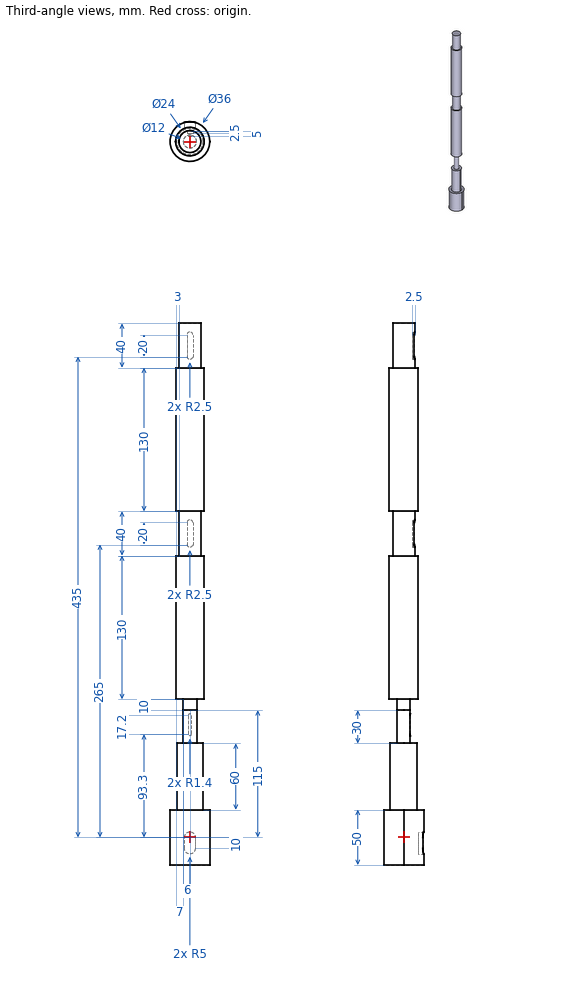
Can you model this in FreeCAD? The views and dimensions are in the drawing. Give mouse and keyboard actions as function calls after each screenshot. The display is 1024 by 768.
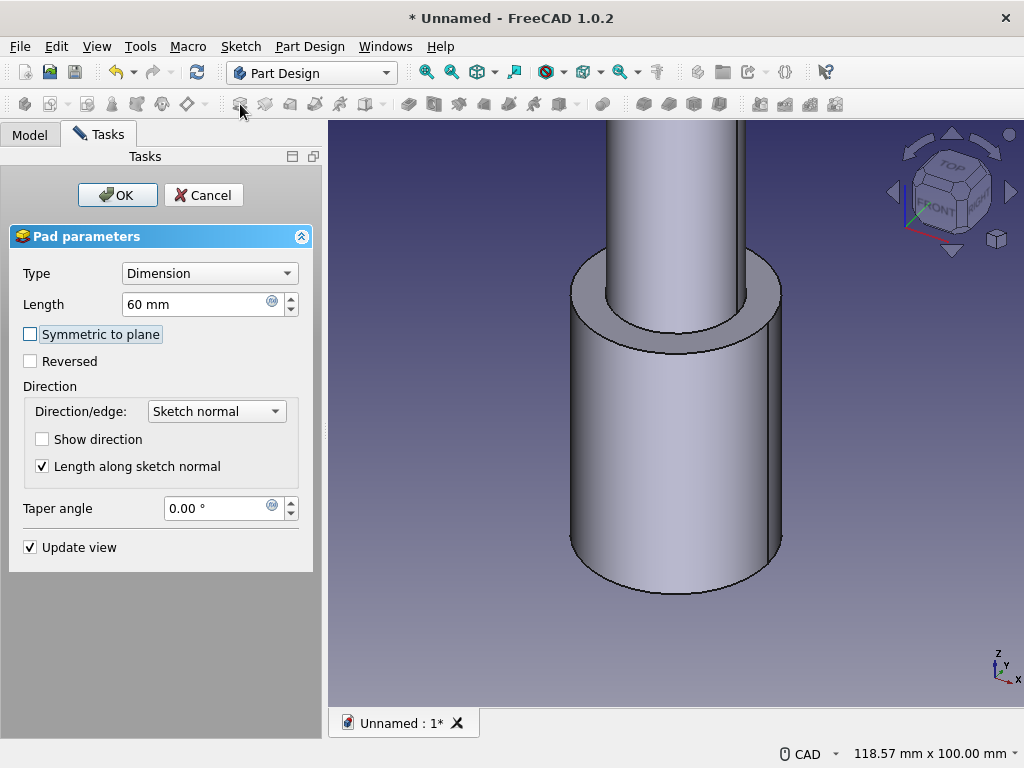
click(118, 195)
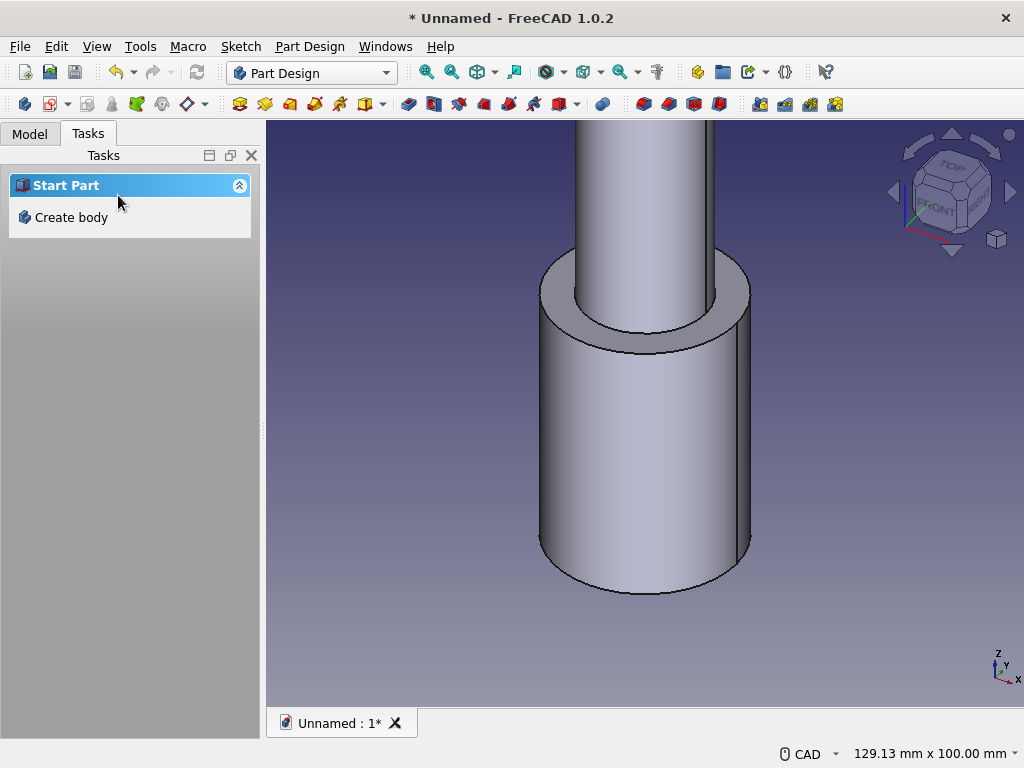
click(427, 72)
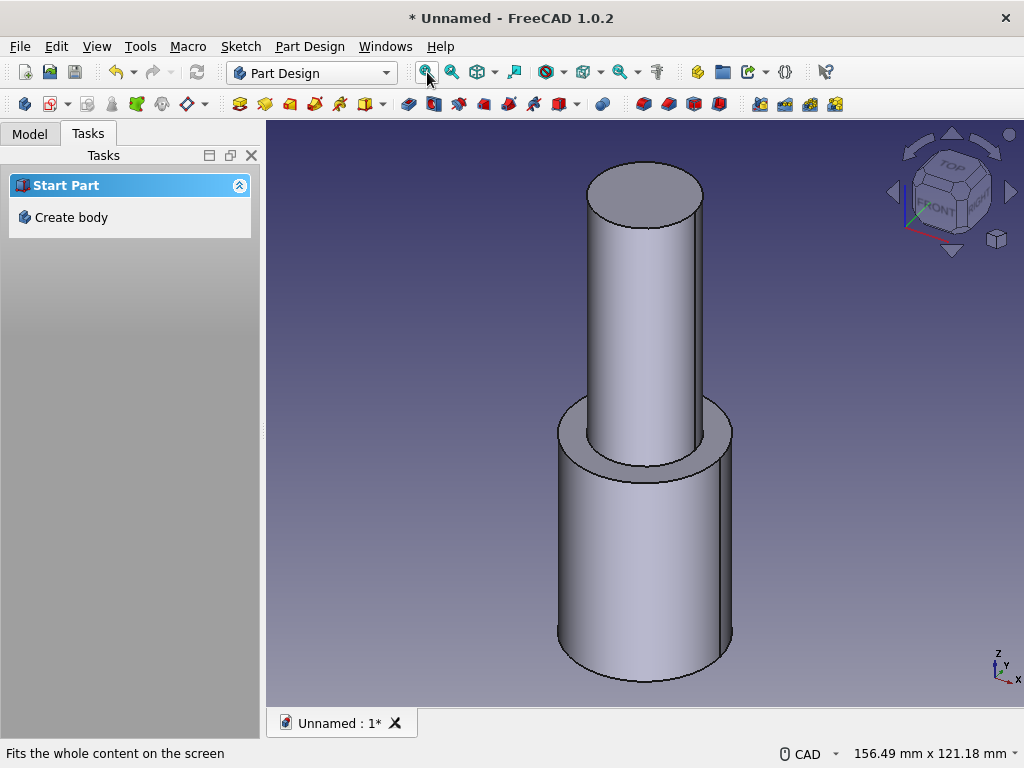
click(645, 194)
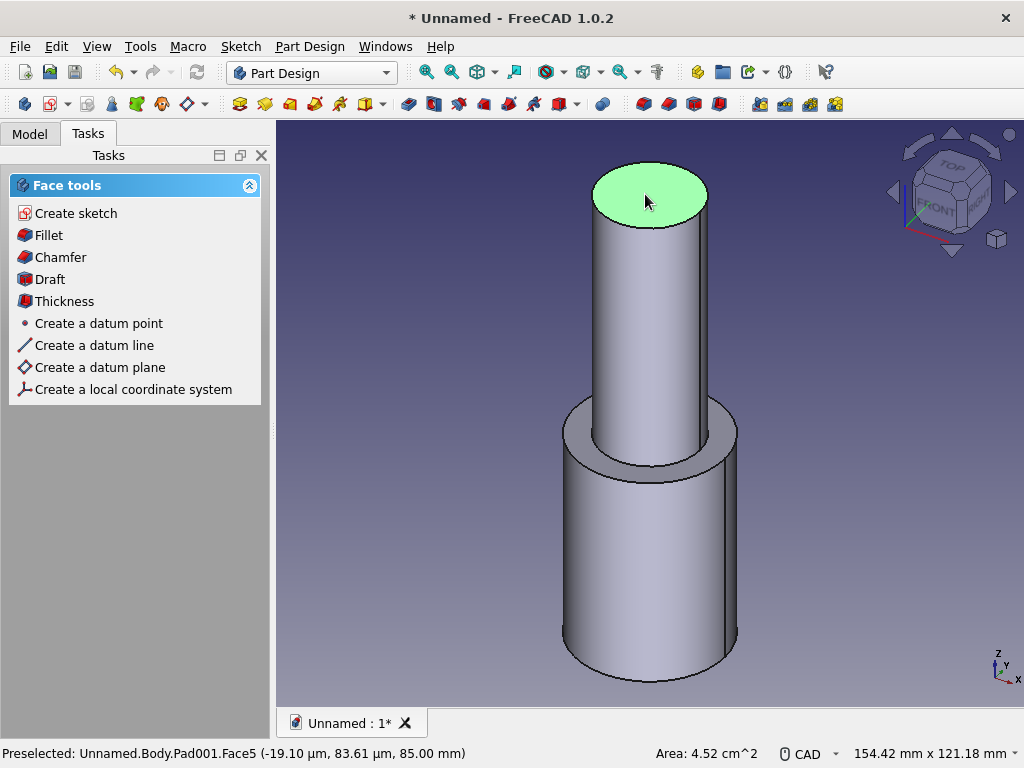
click(50, 104)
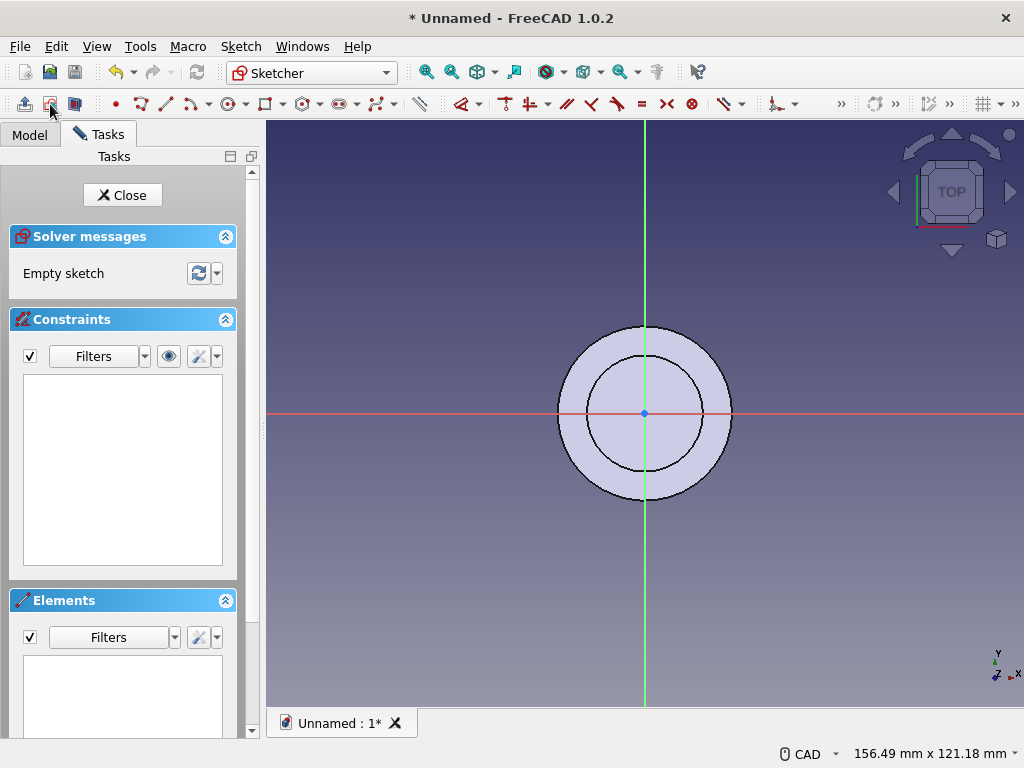
scroll(658, 414, up, 9)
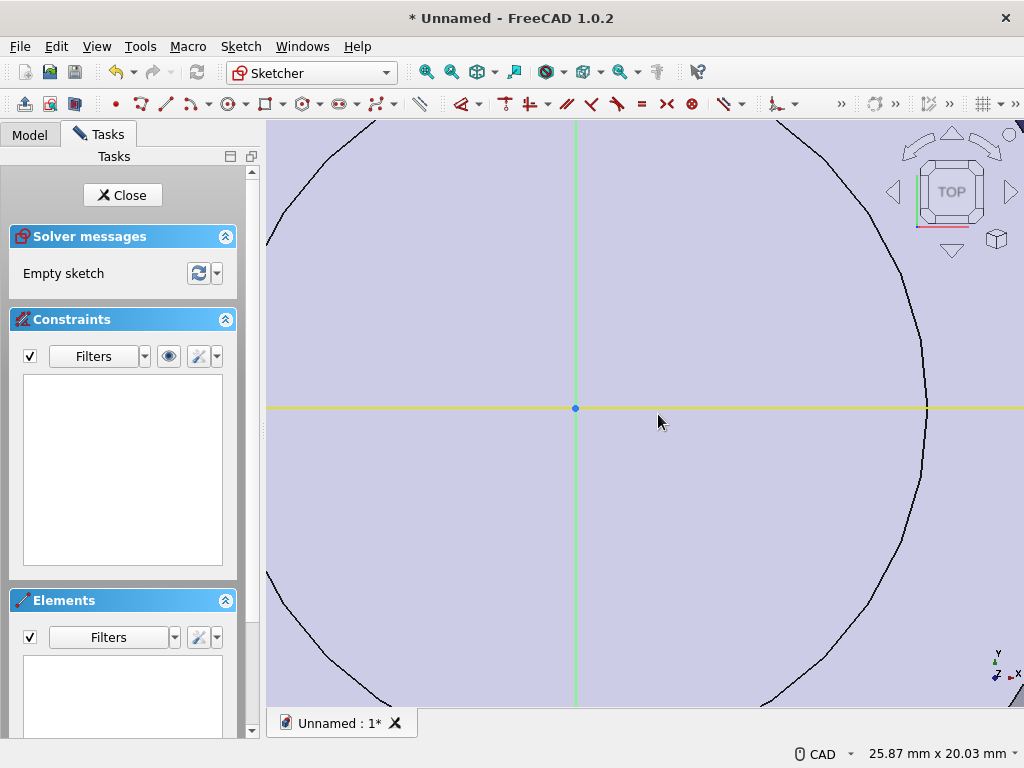
click(228, 104)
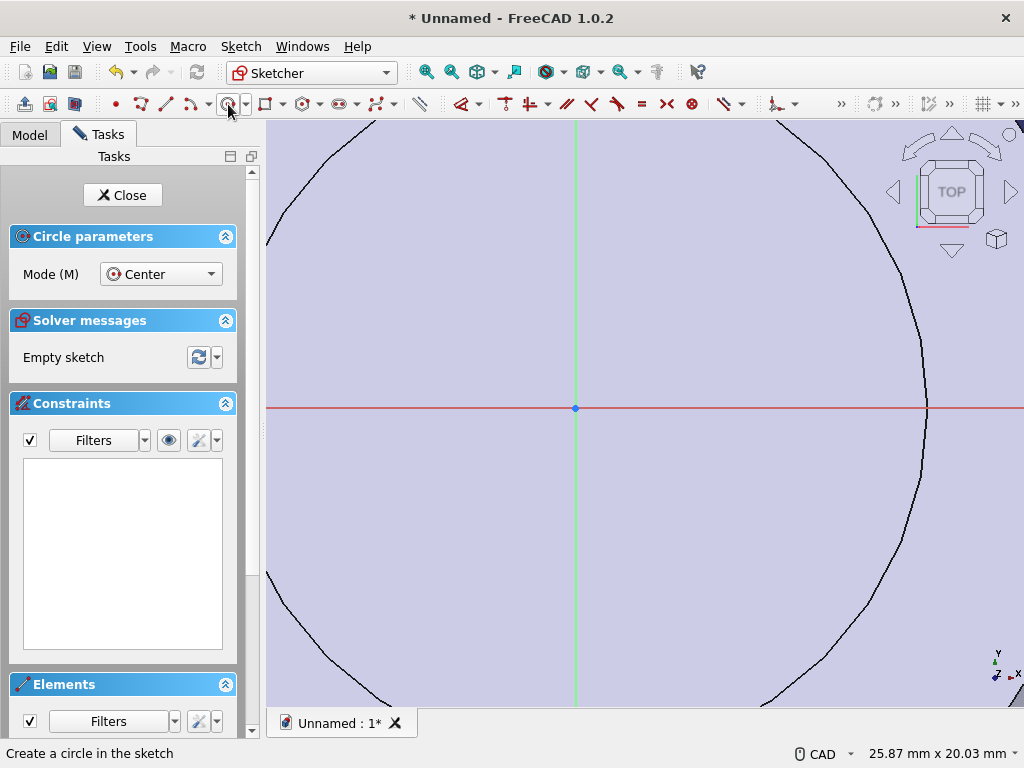
click(576, 408)
click(700, 284)
key(Escape)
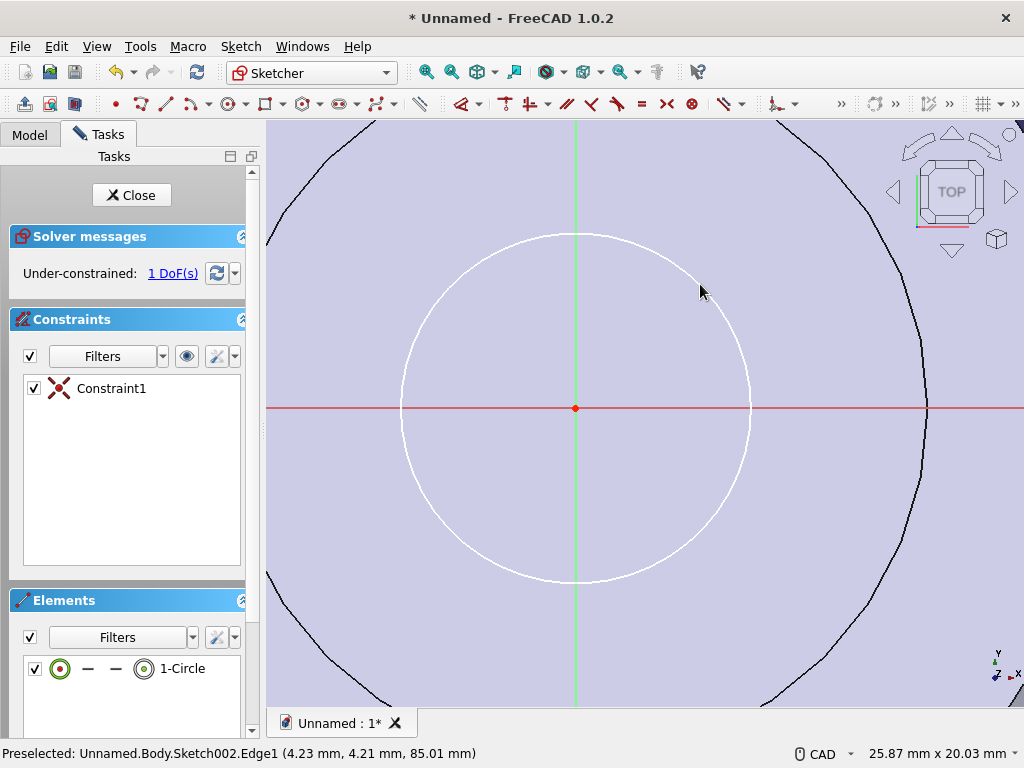
click(460, 104)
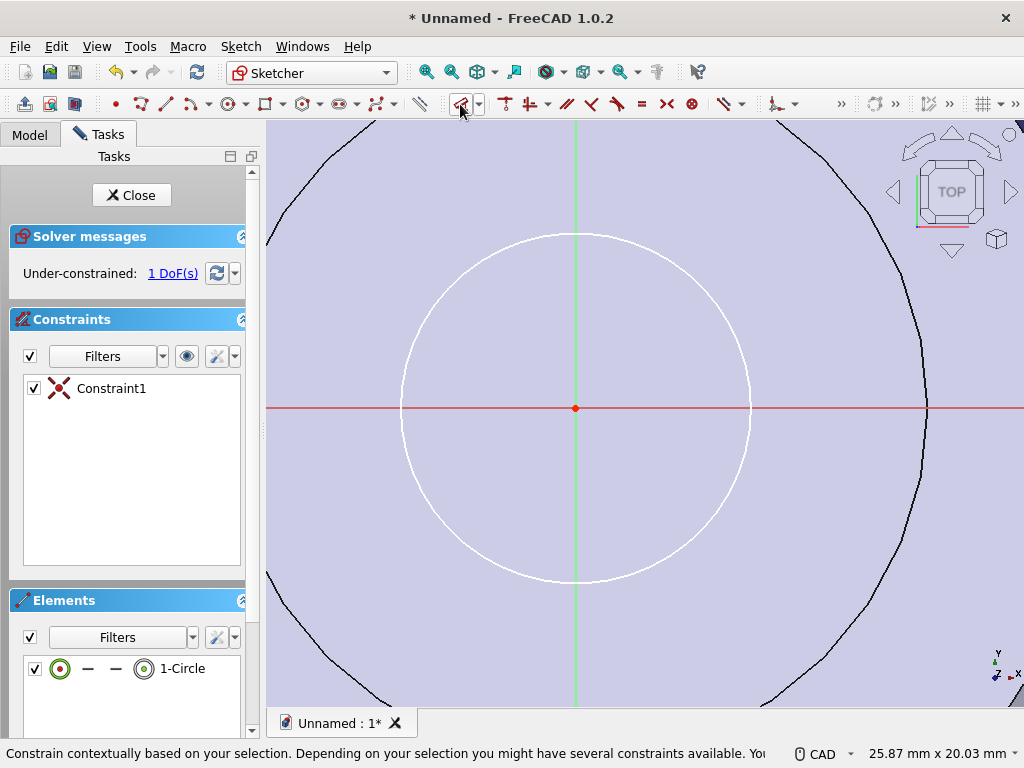
click(699, 284)
click(722, 261)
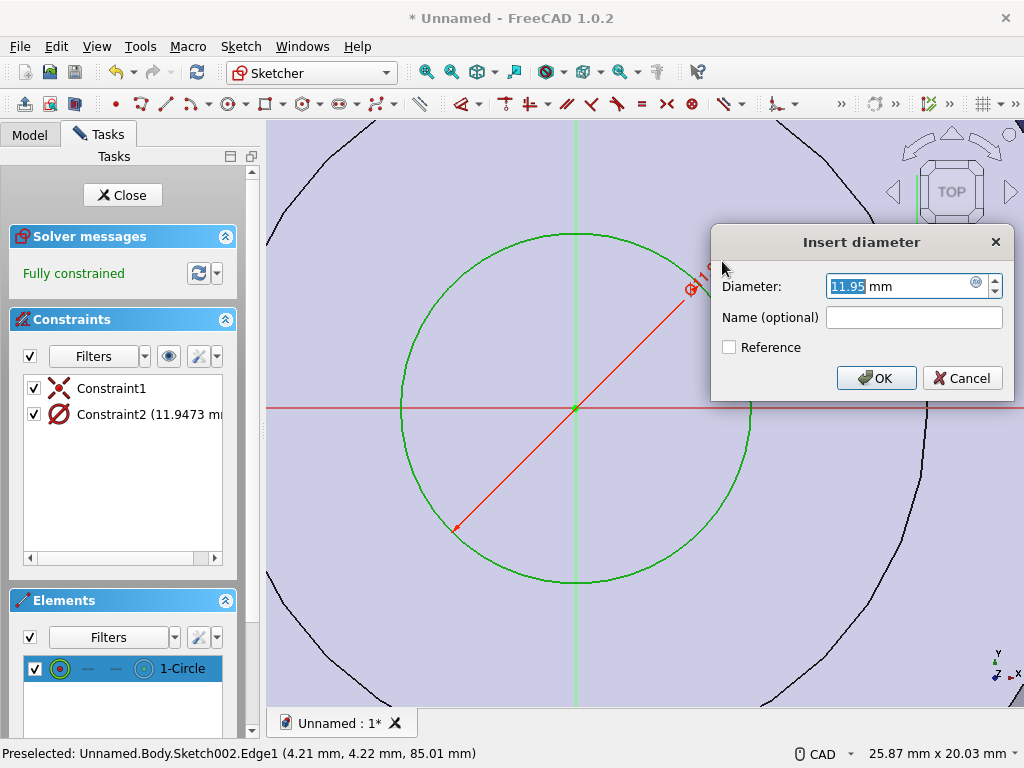
text(12)
key(Return)
key(Escape)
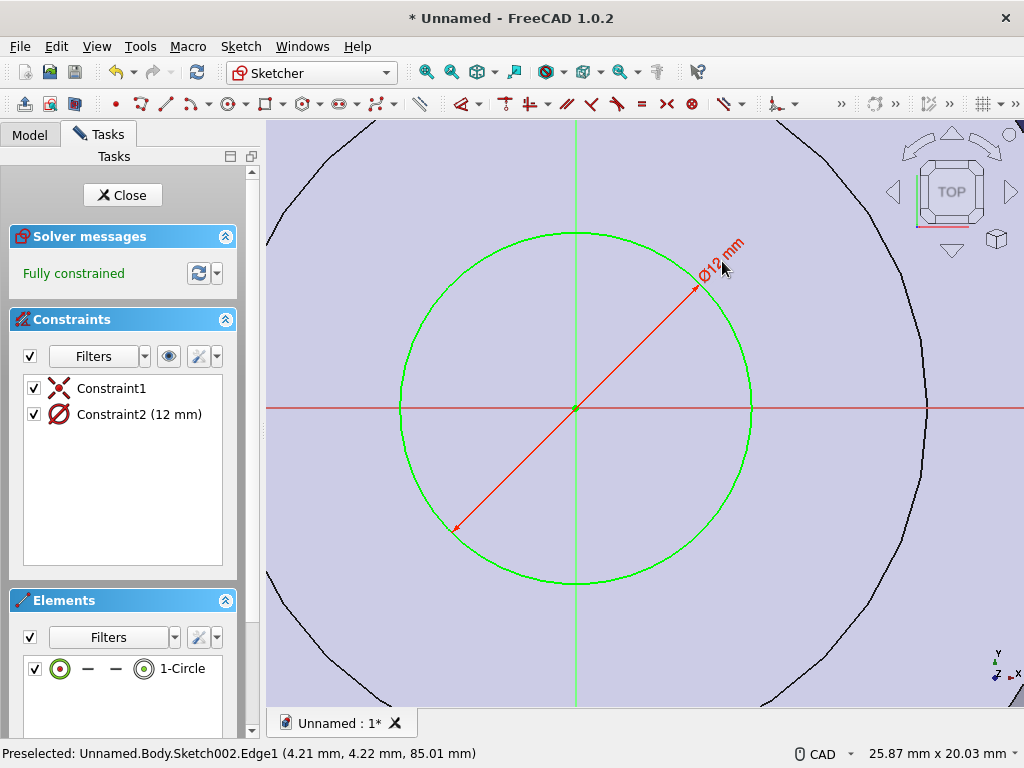
click(123, 195)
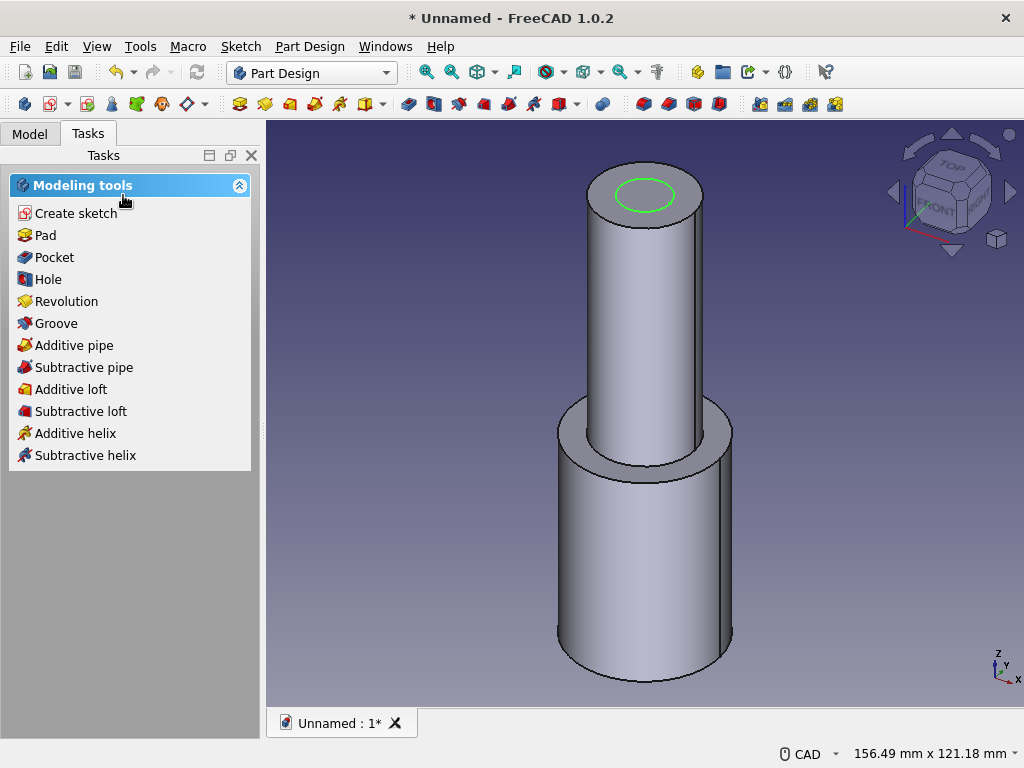
click(240, 104)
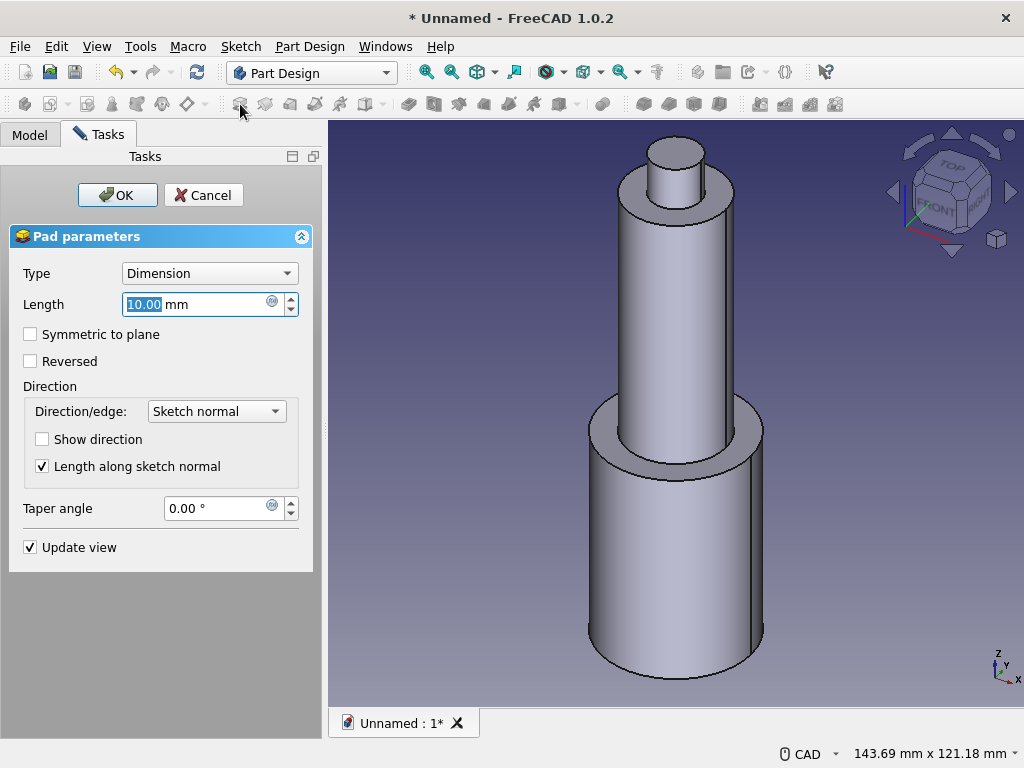
text(30)
key(Tab)